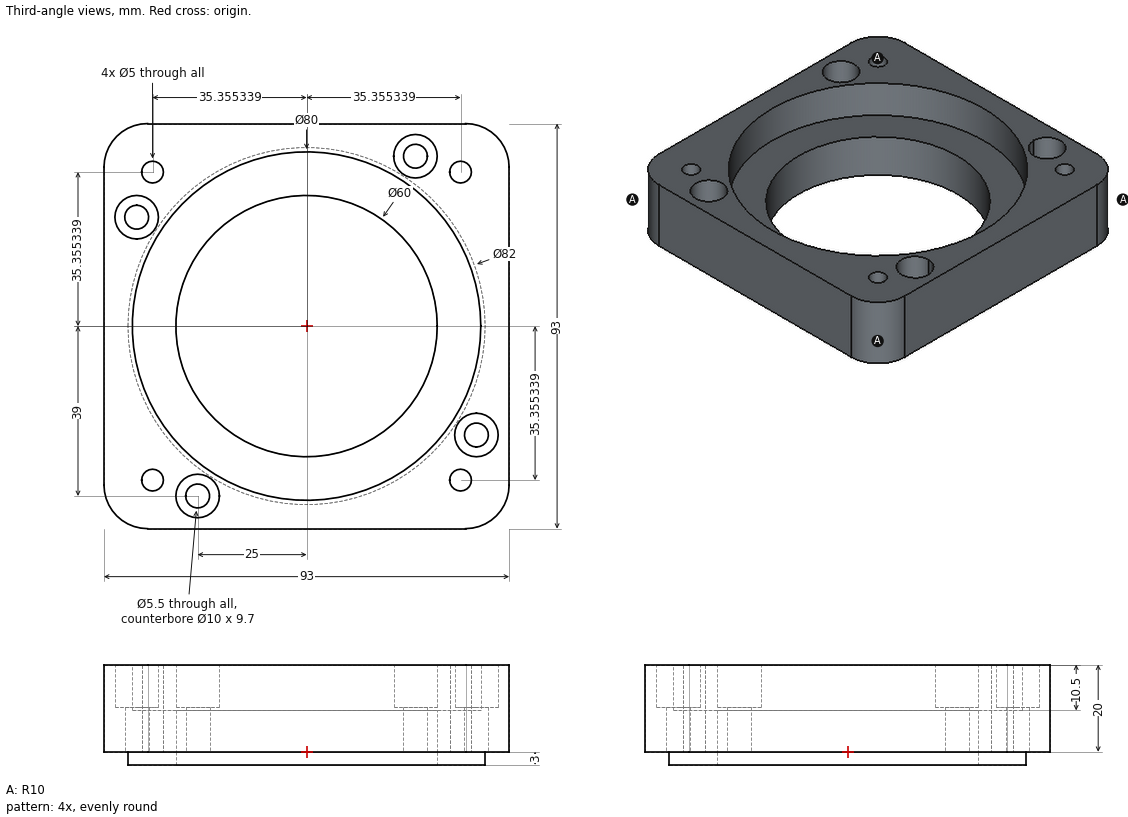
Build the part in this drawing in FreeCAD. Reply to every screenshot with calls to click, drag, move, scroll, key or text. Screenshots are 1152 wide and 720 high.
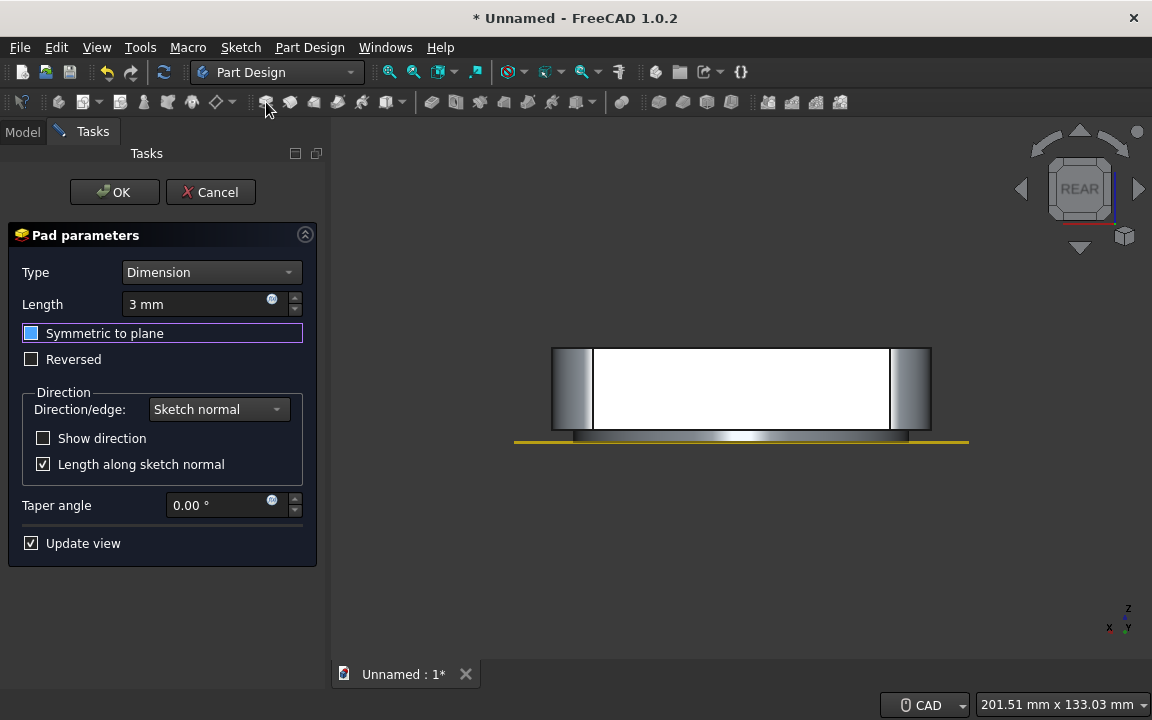
click(115, 192)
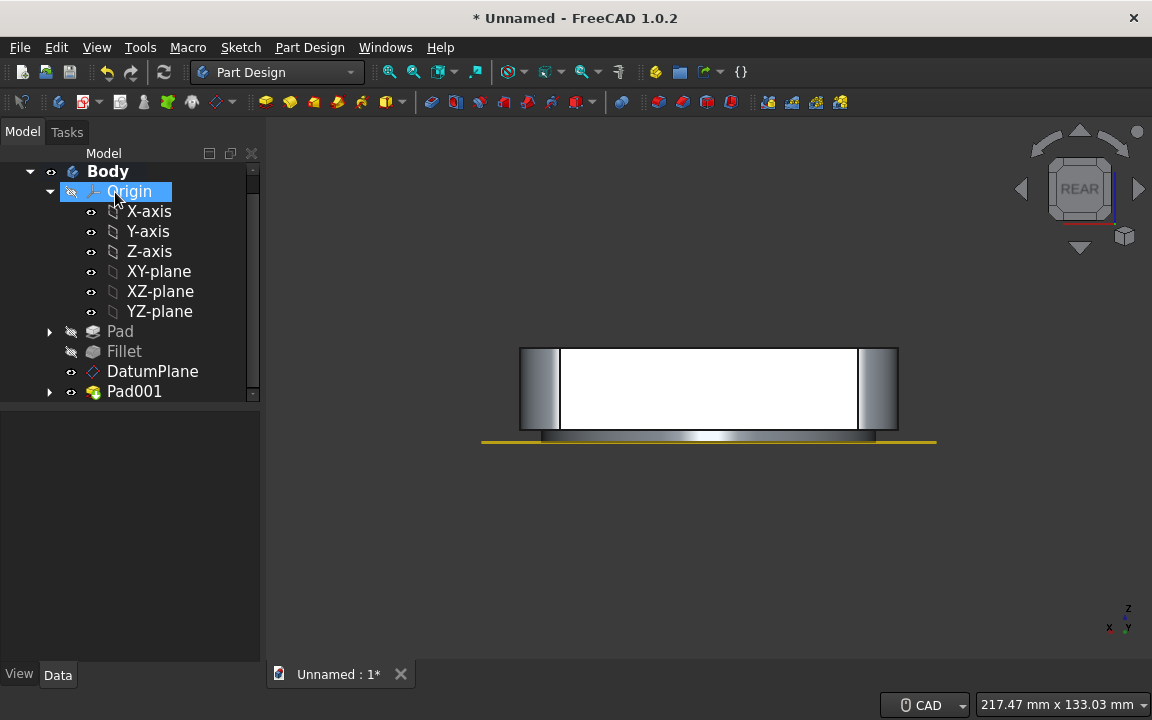
click(116, 372)
key(space)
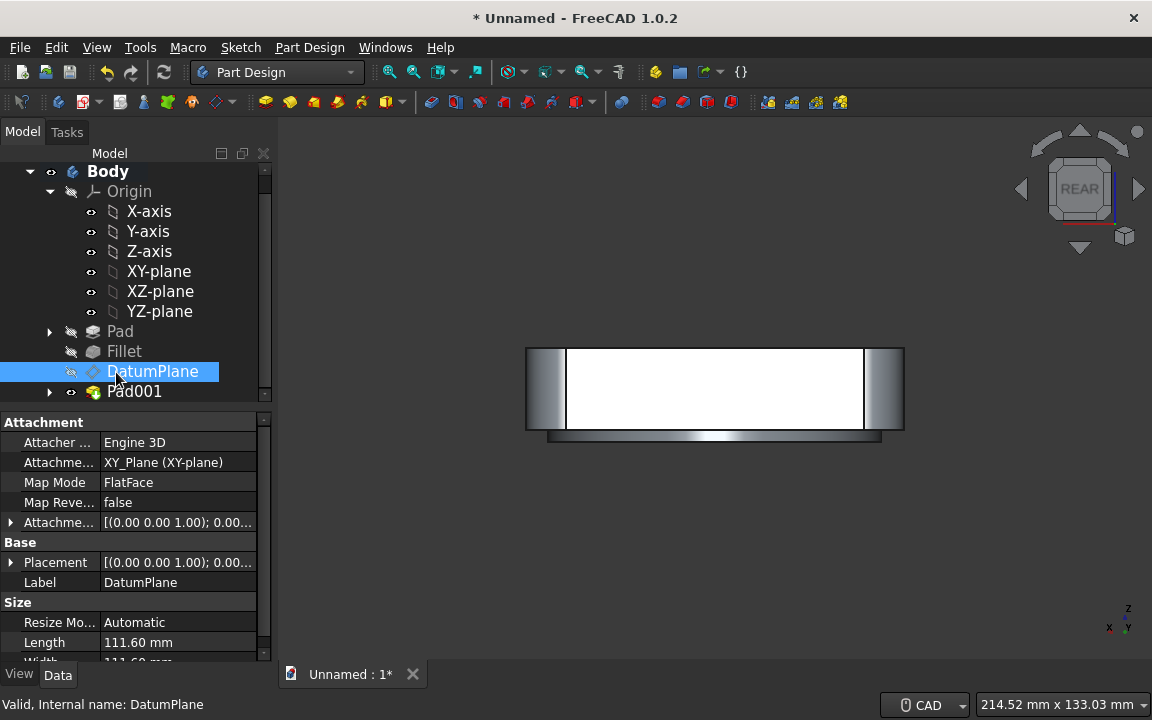
click(390, 72)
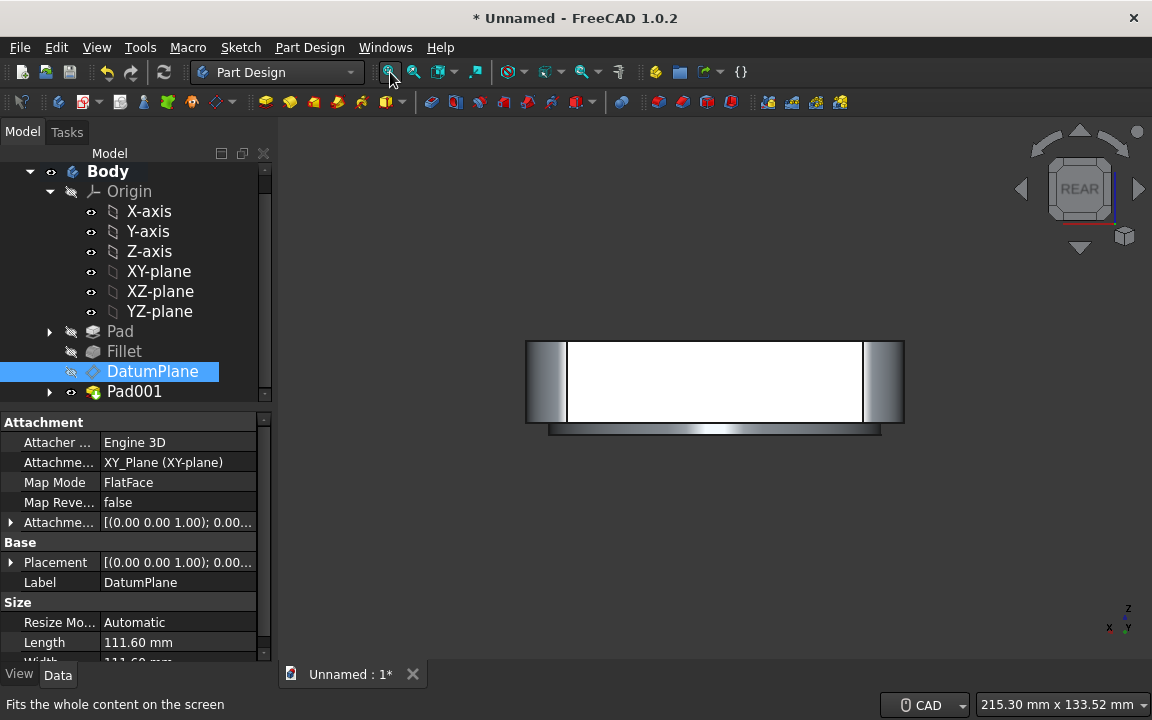
key(0)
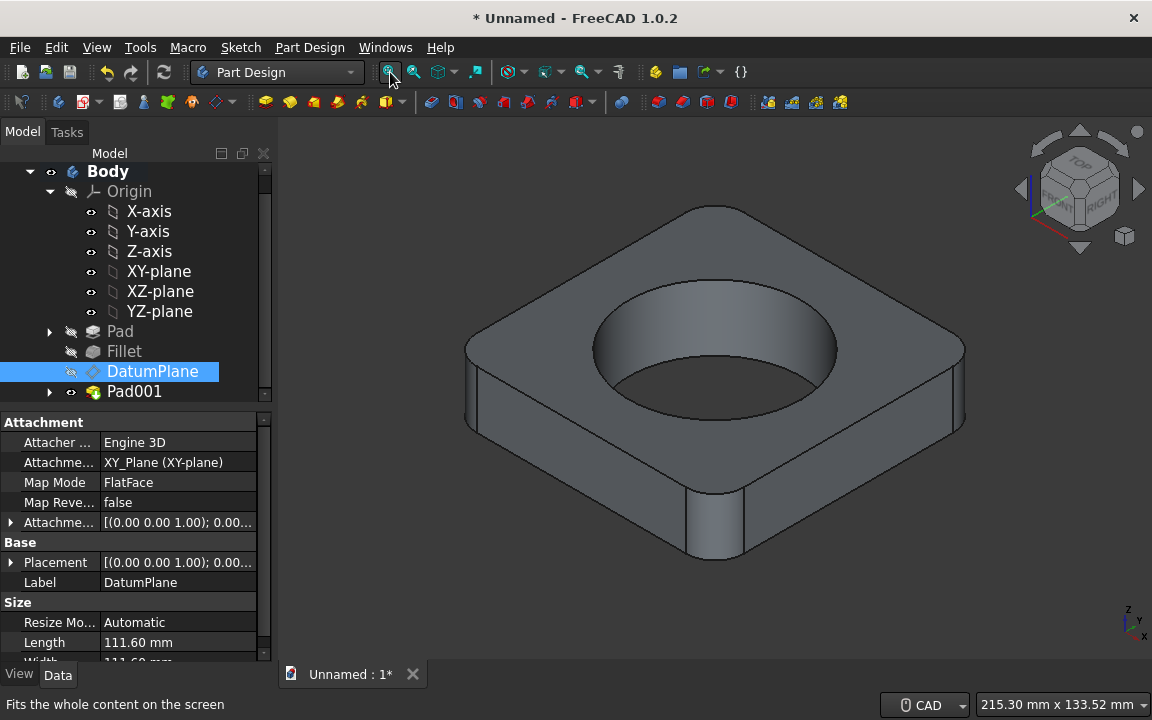
click(715, 437)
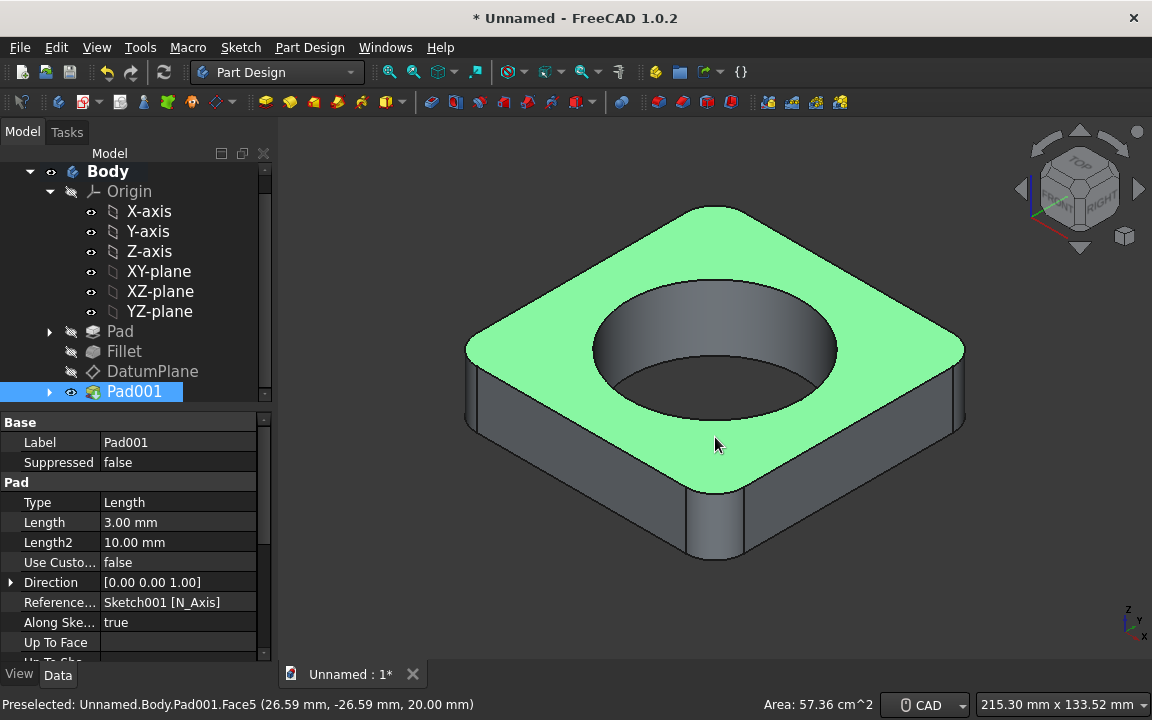
click(84, 102)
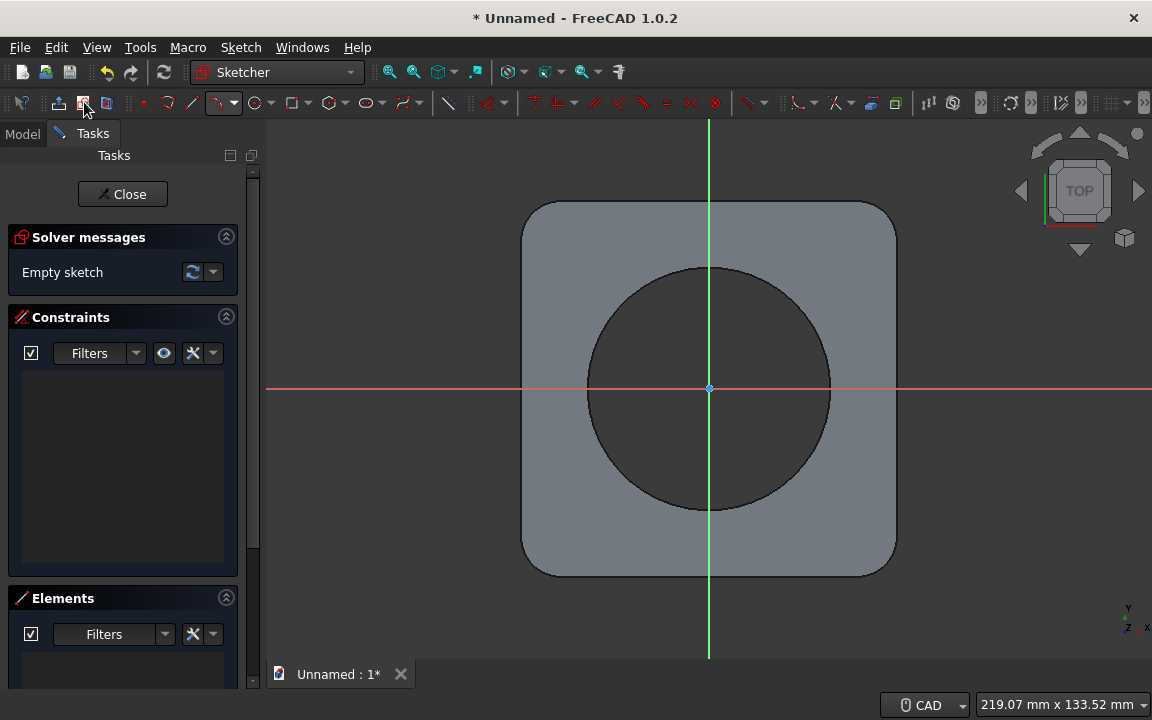
click(256, 104)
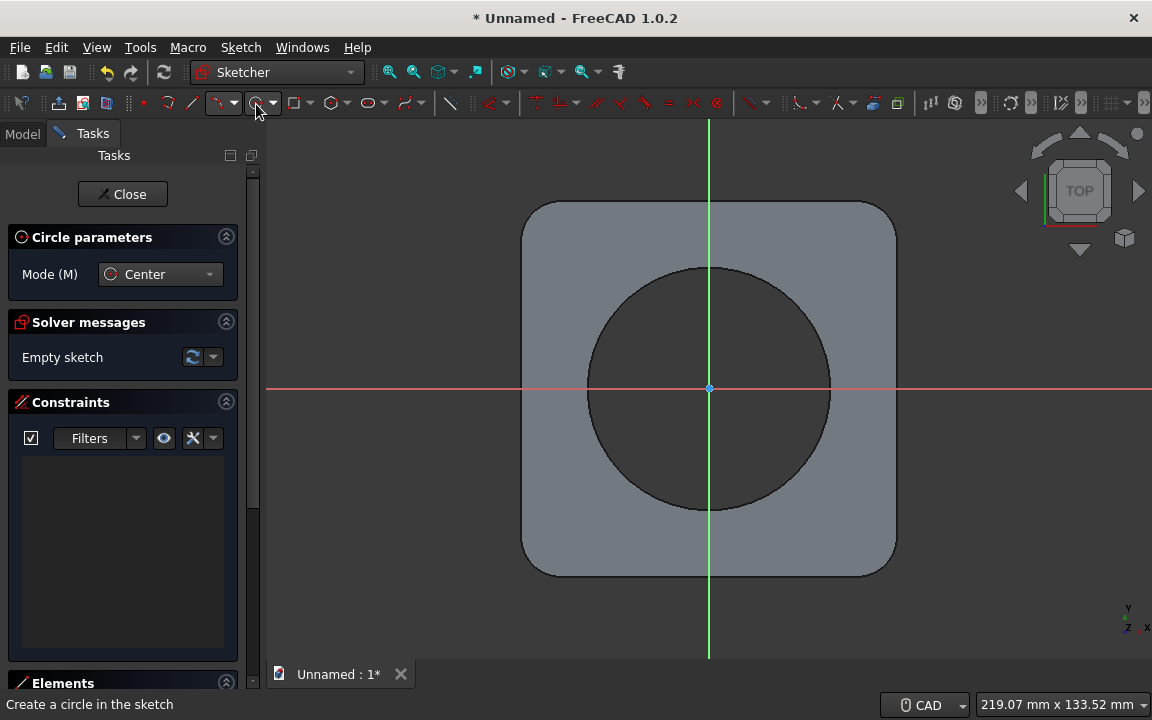
click(709, 389)
click(823, 275)
key(Escape)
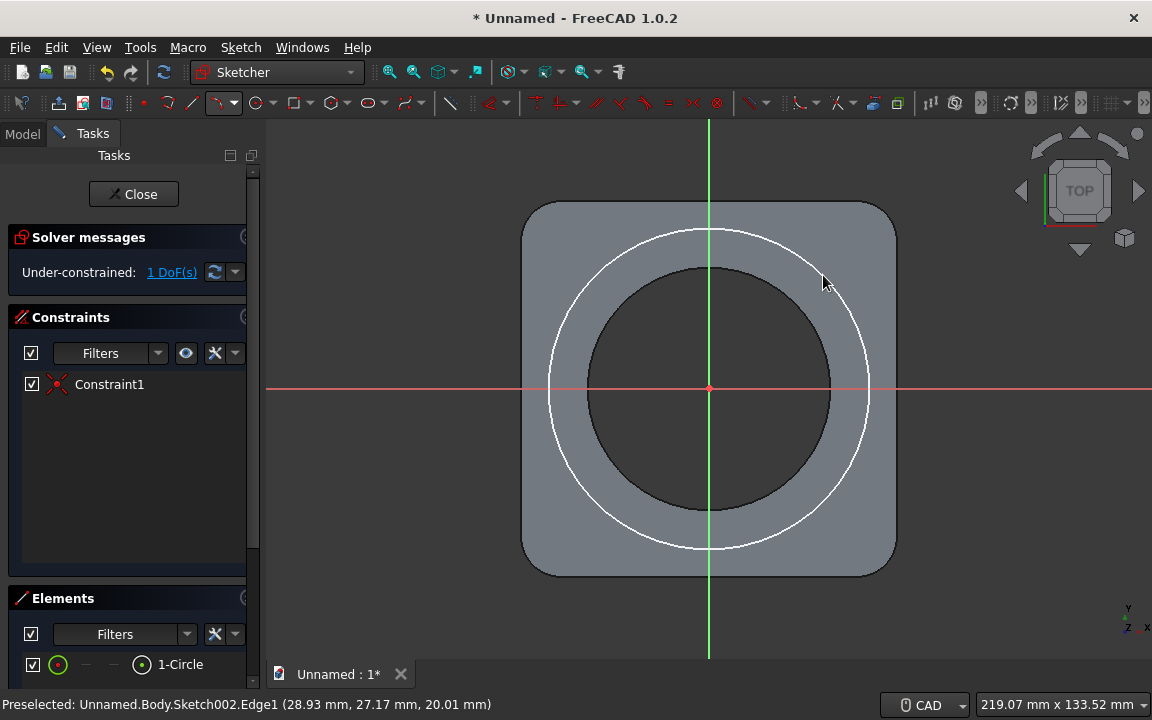
click(490, 104)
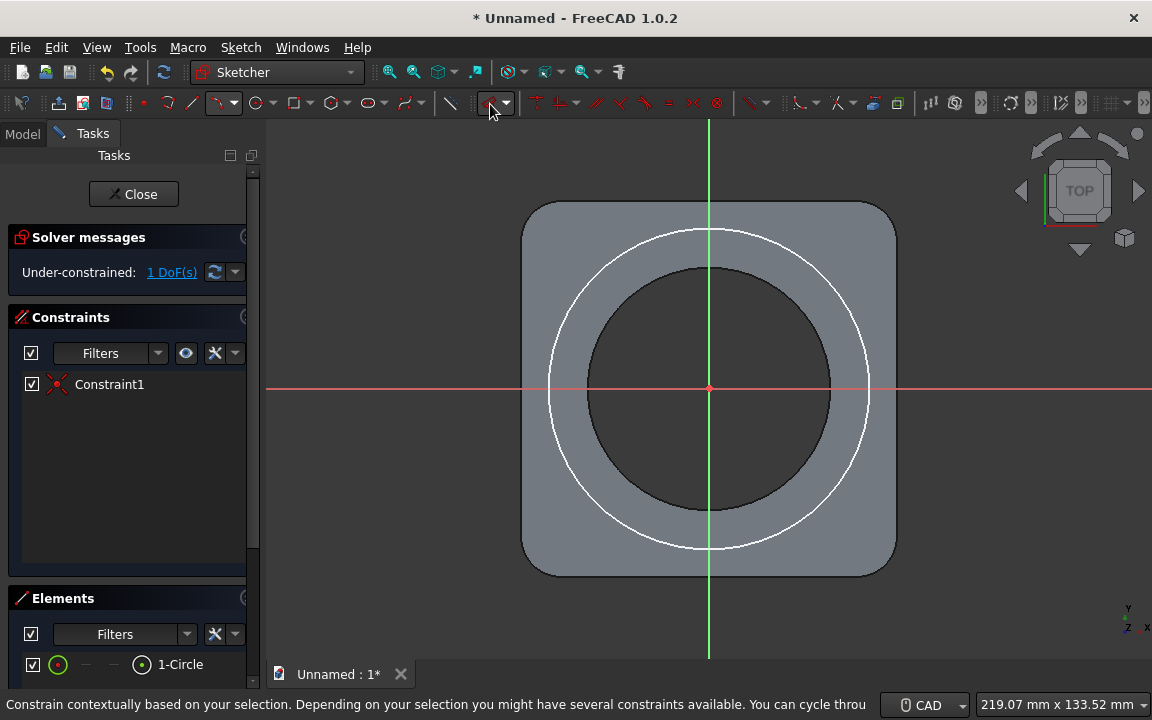
click(822, 275)
click(845, 252)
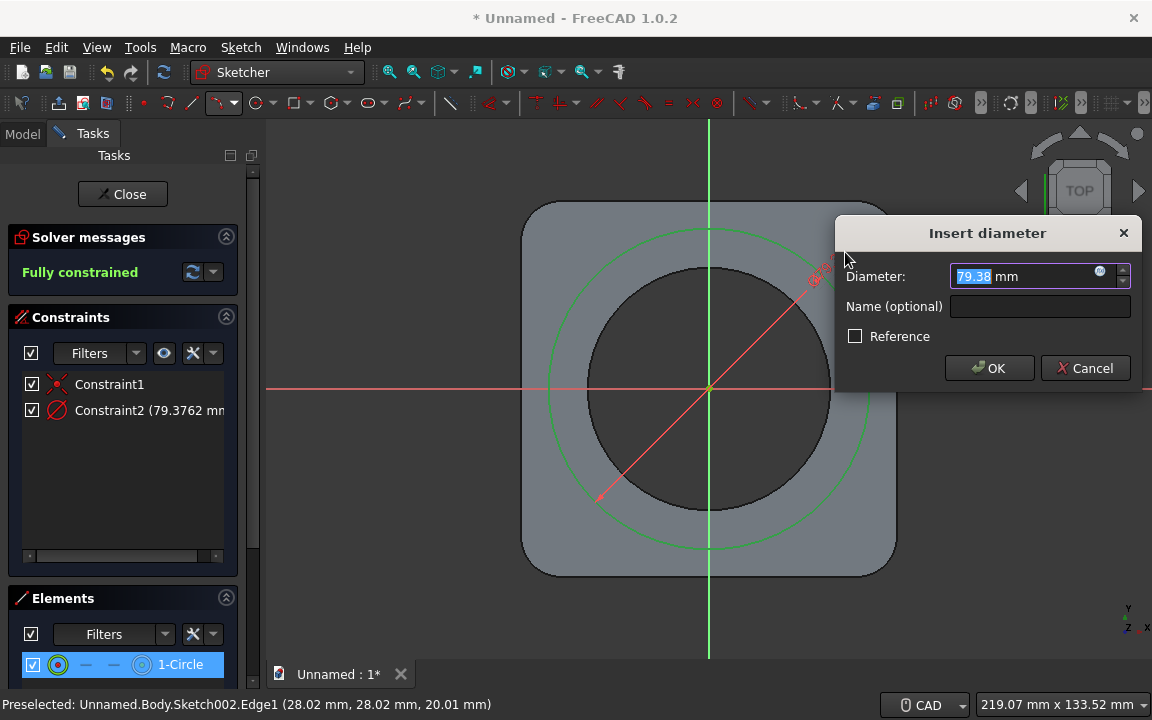
text(80)
key(Return)
key(Escape)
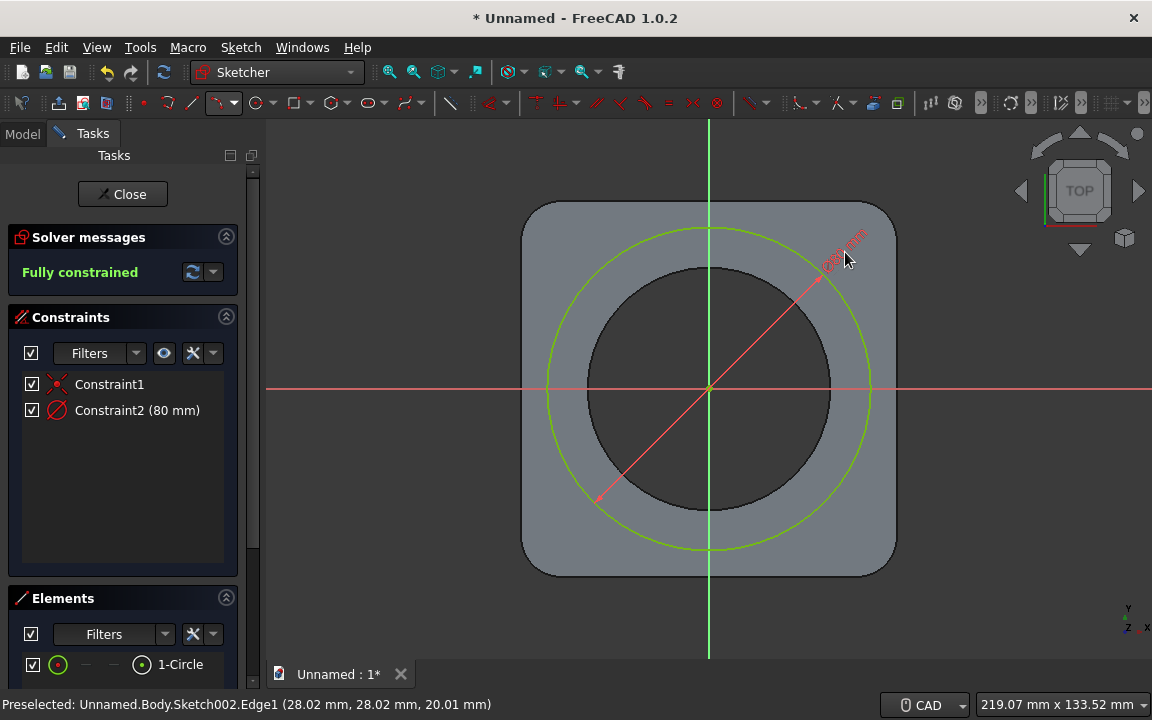
click(123, 194)